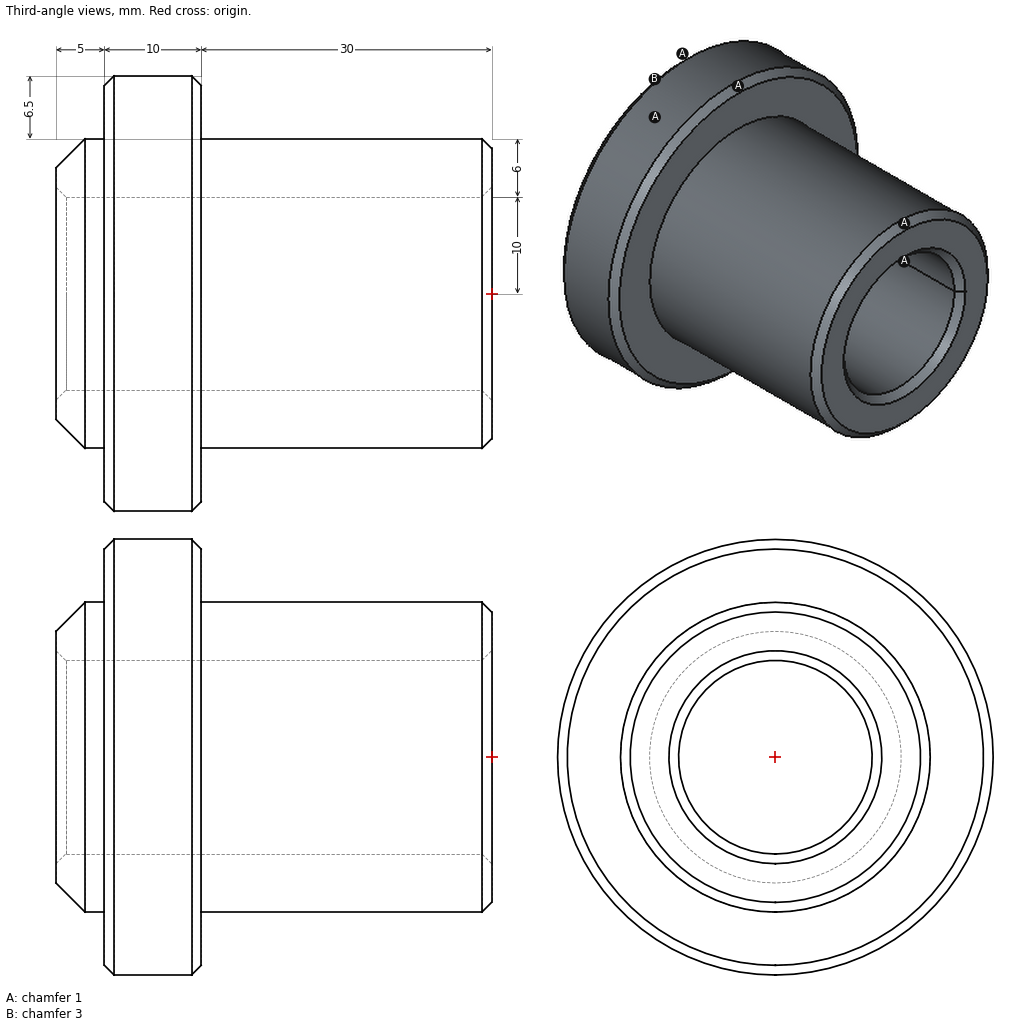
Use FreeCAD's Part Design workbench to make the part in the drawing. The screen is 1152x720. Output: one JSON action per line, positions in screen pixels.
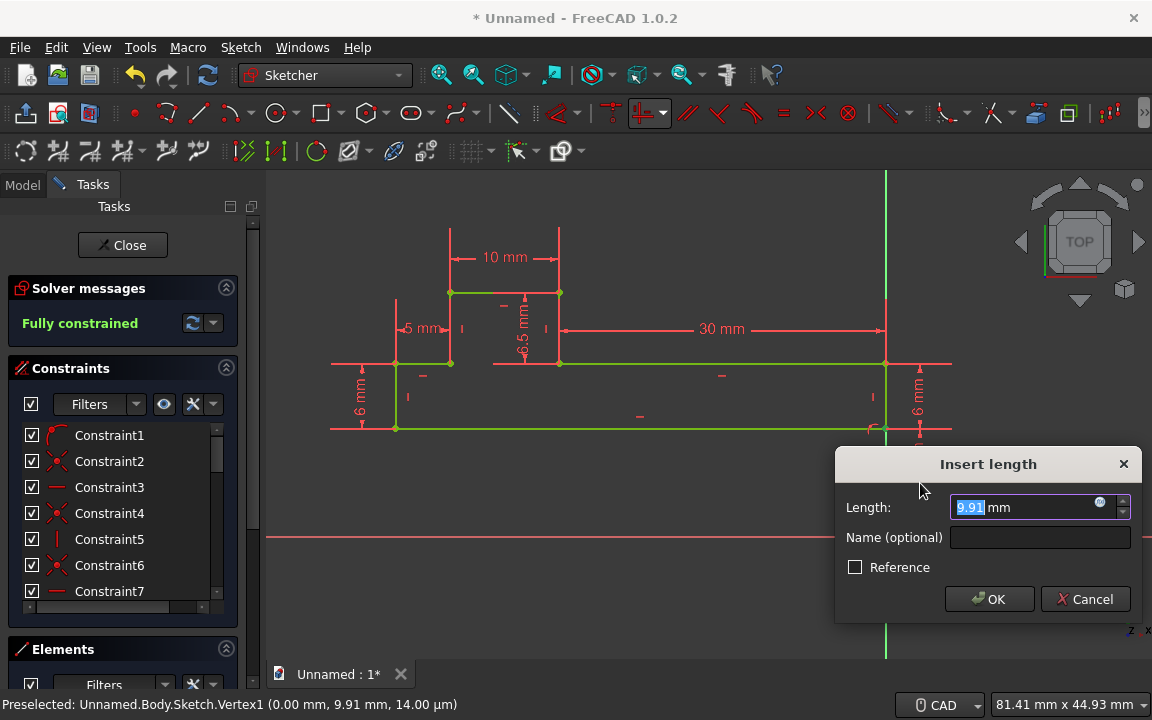
{"action": "type", "text": "10"}
{"action": "key", "text": "Return"}
{"action": "key", "text": "Escape"}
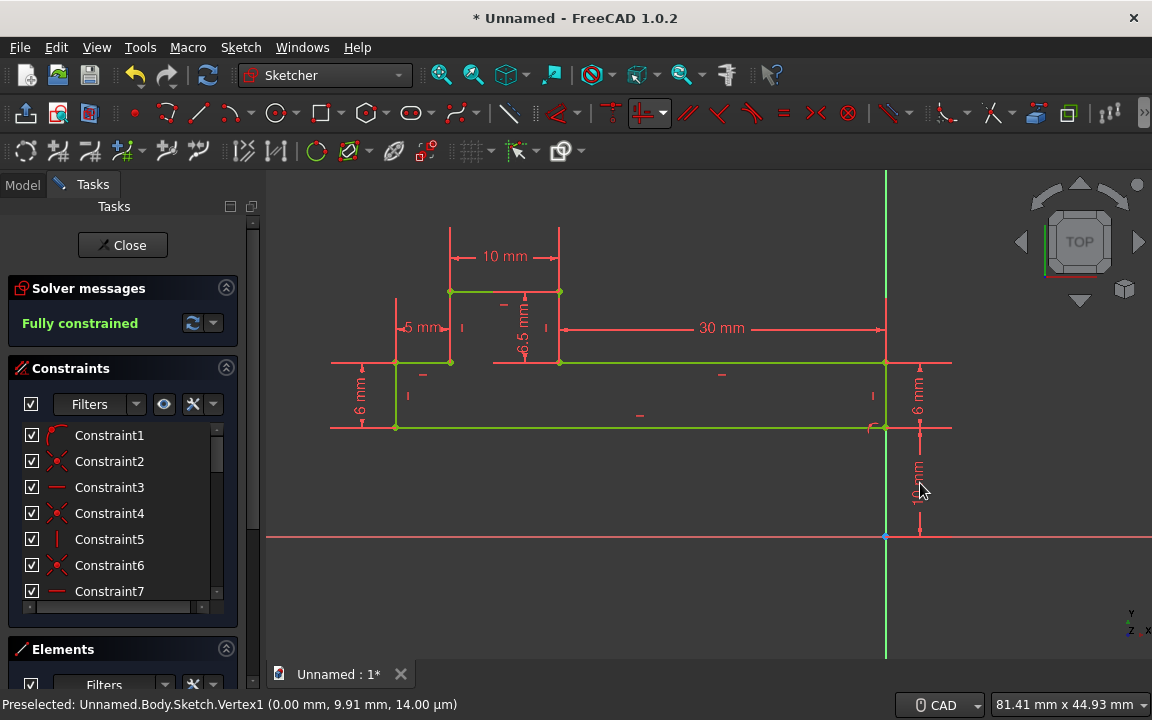
{"action": "left_click", "coordinate": [123, 245]}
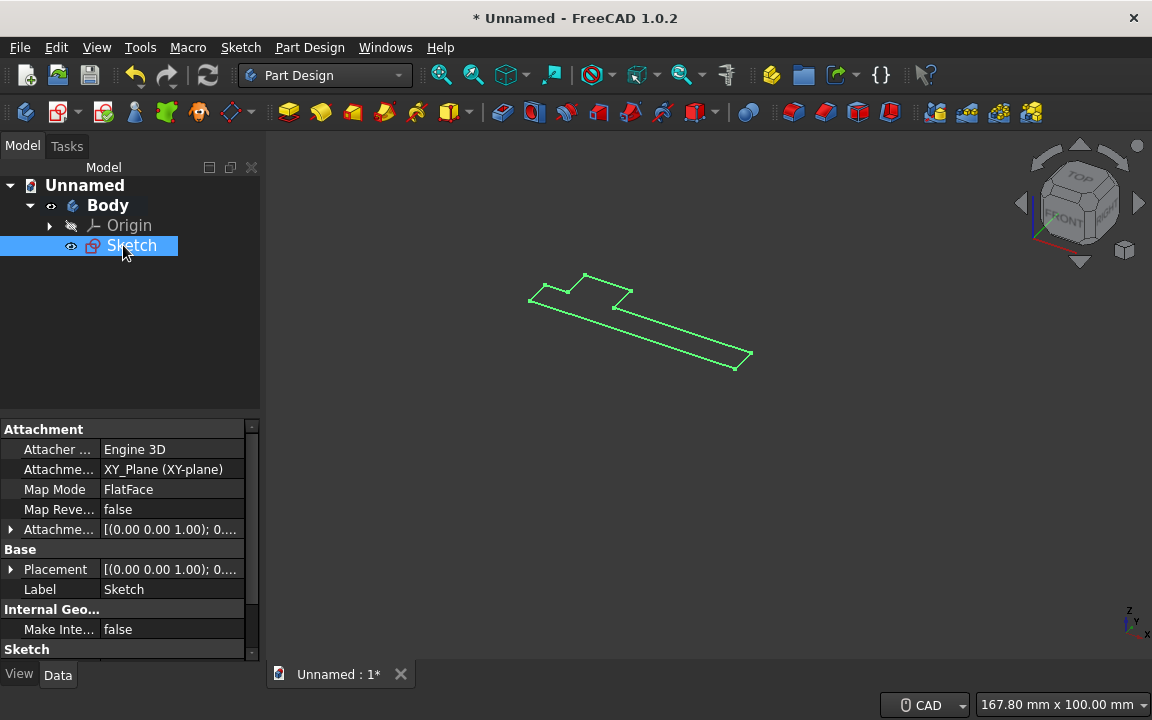
{"action": "left_click", "coordinate": [322, 112]}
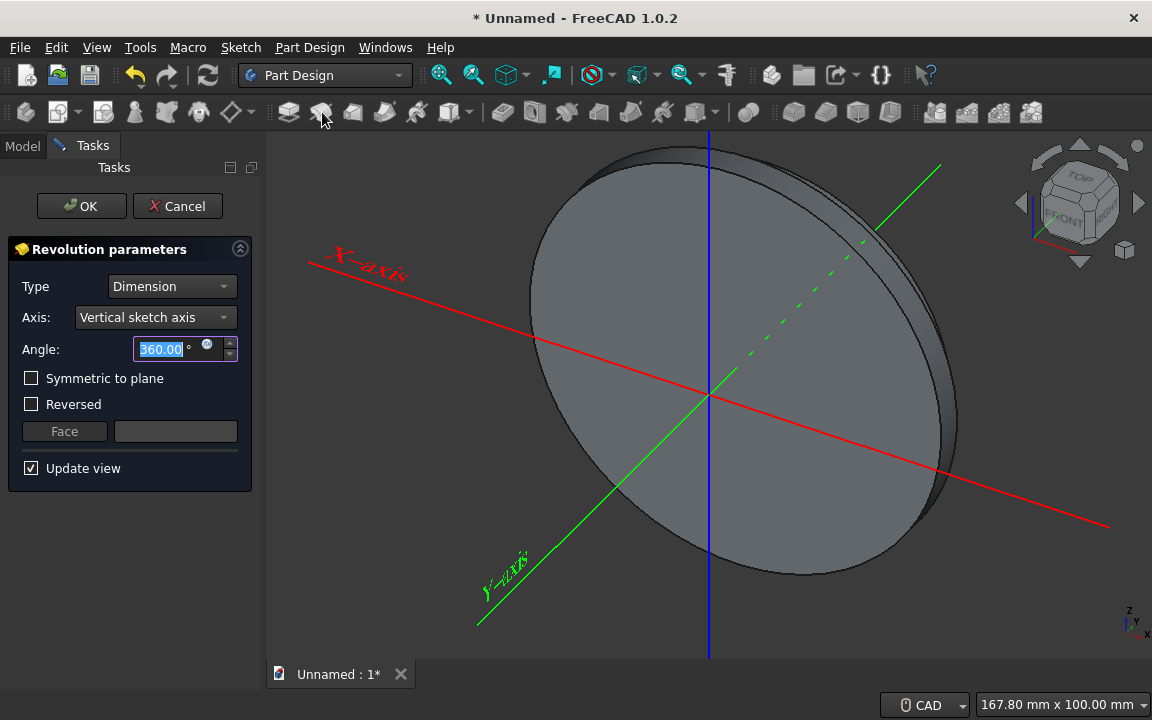
{"action": "left_click", "coordinate": [156, 318]}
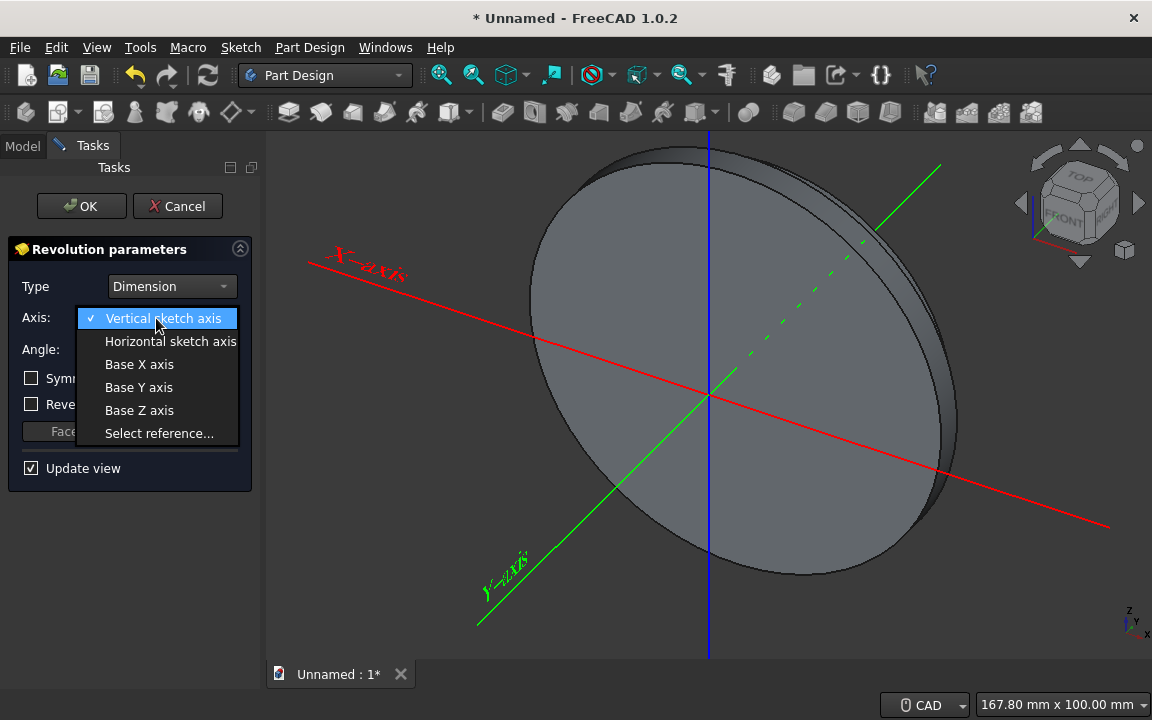
{"action": "left_click", "coordinate": [156, 342]}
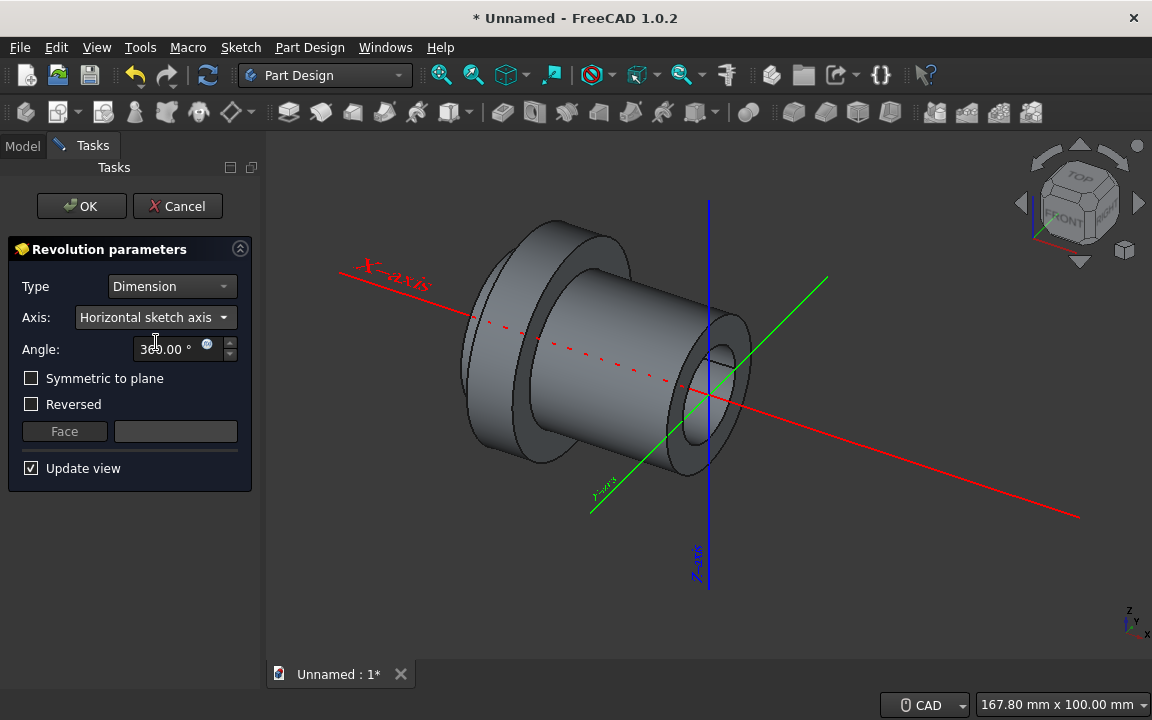
{"action": "left_click", "coordinate": [82, 206]}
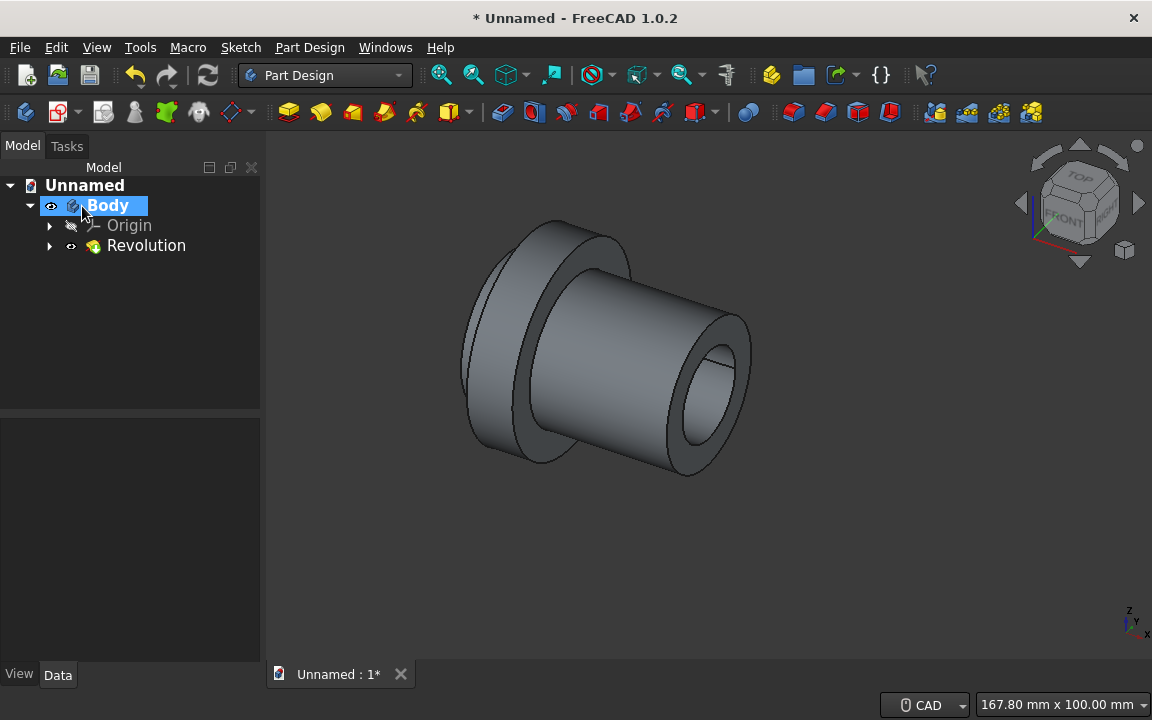
{"action": "left_click", "coordinate": [667, 436]}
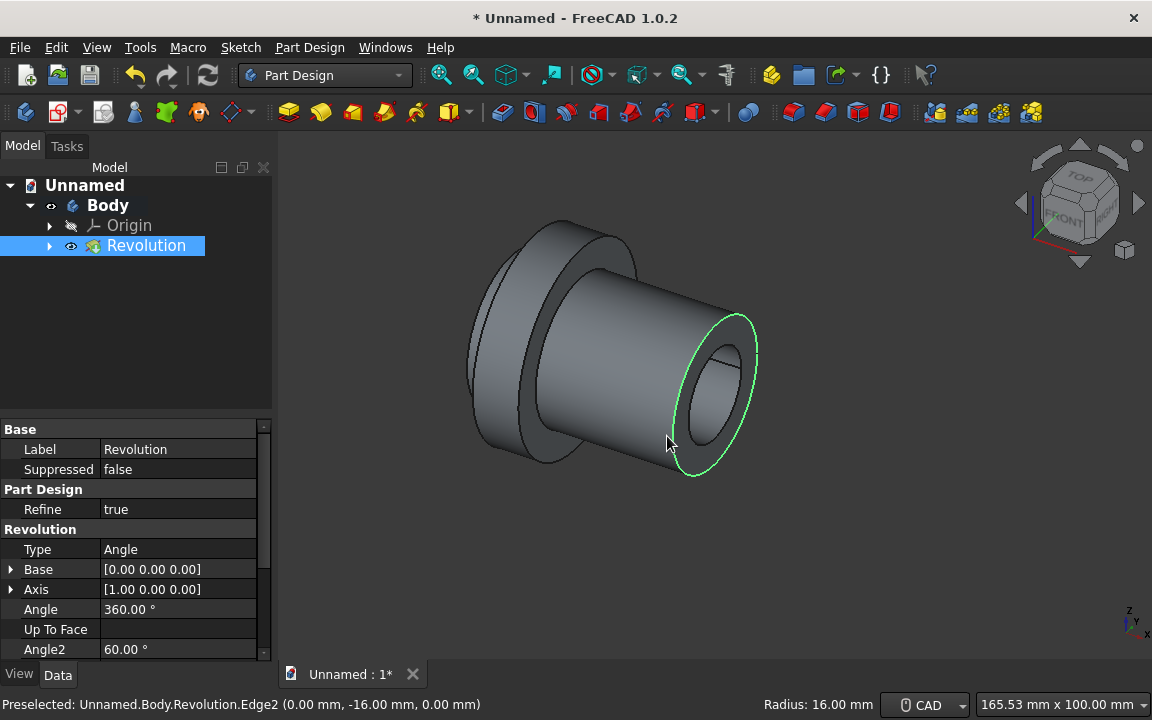
{"action": "left_click", "coordinate": [518, 408], "text": "ctrl"}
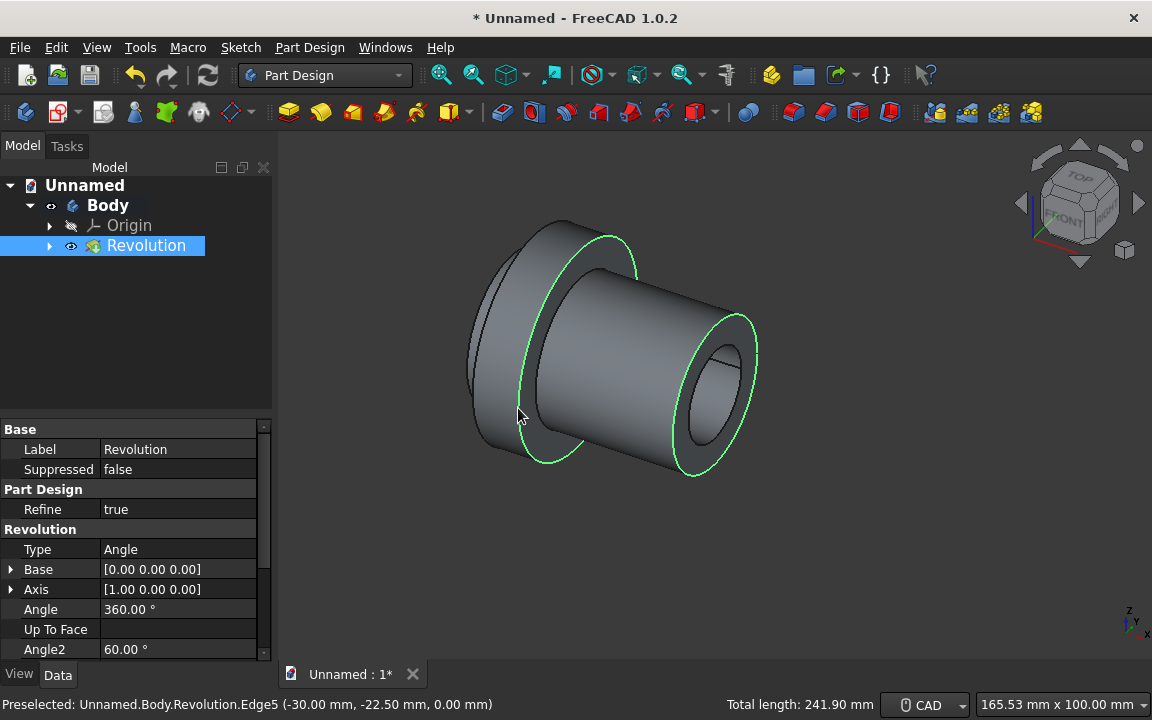
{"action": "left_click", "coordinate": [707, 443], "text": "ctrl"}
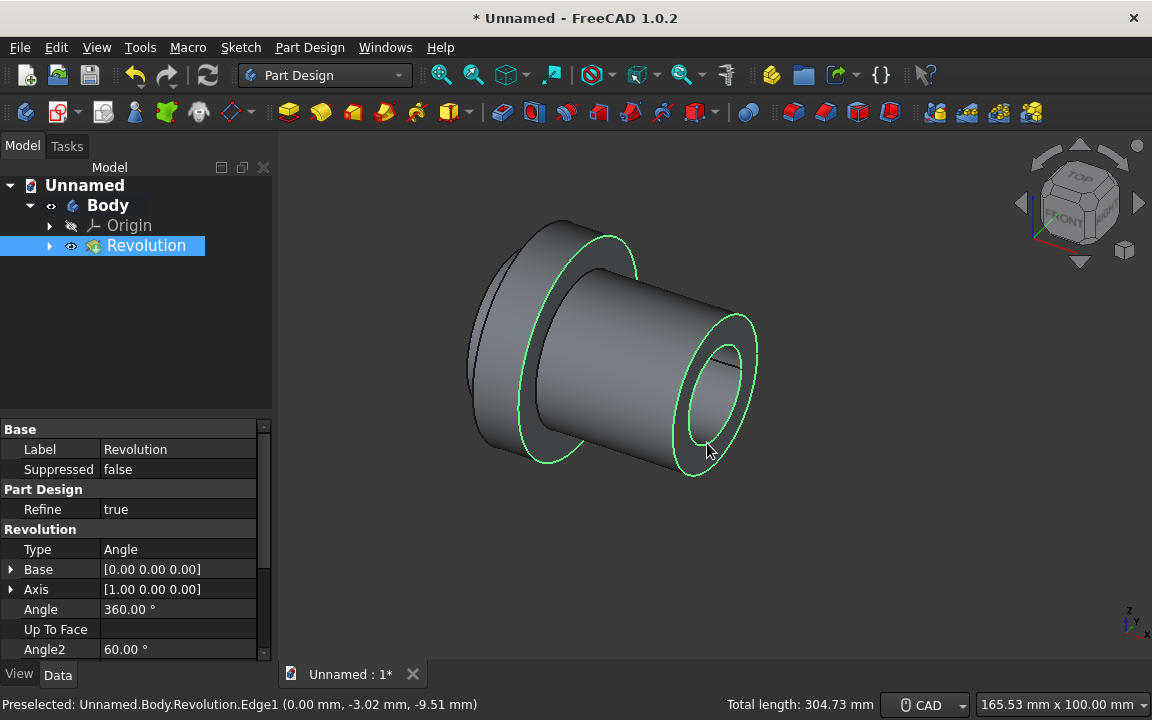
{"action": "key", "text": "0"}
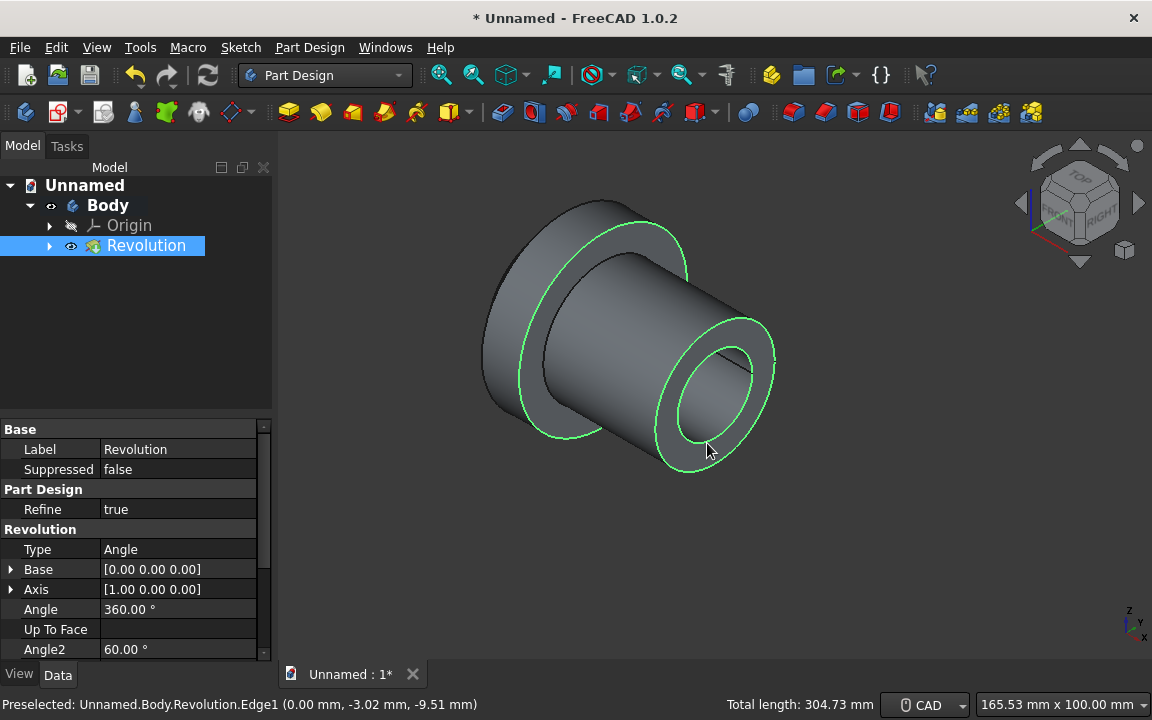
{"action": "key", "text": "2"}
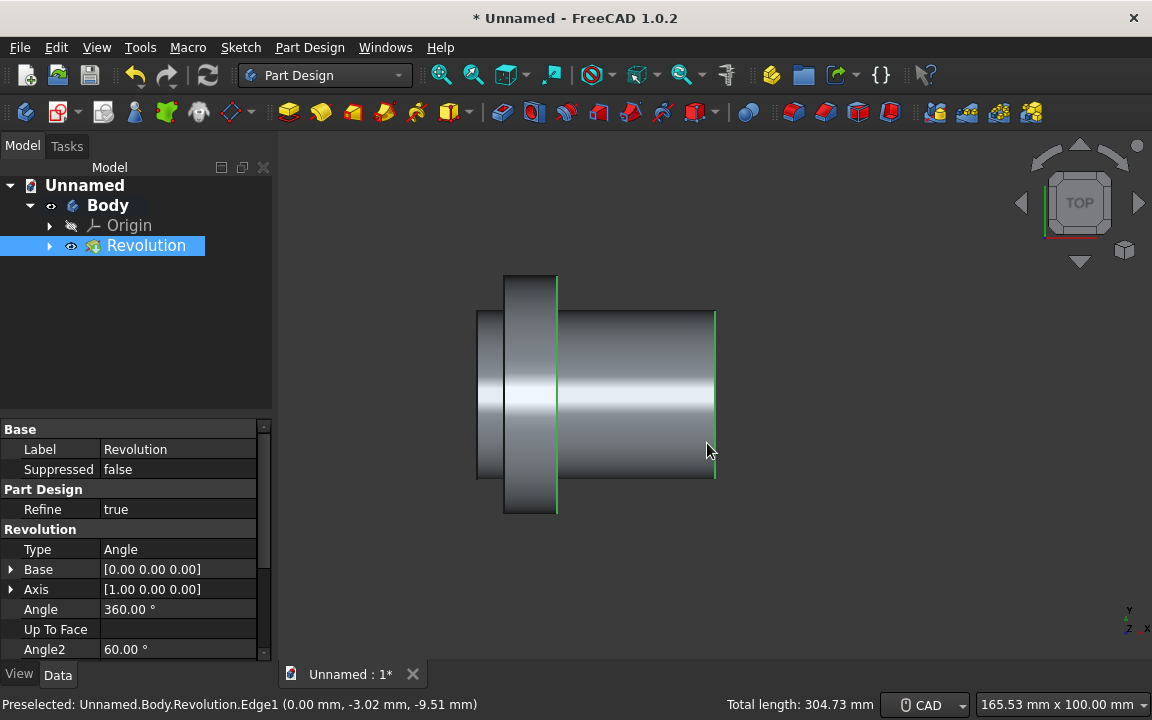
{"action": "left_click", "coordinate": [504, 490], "text": "ctrl"}